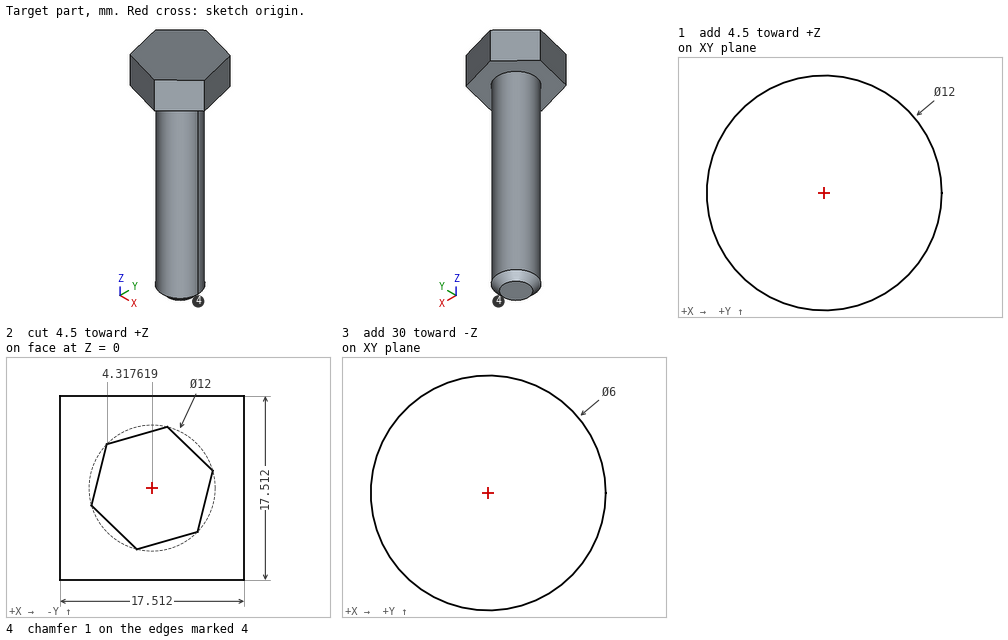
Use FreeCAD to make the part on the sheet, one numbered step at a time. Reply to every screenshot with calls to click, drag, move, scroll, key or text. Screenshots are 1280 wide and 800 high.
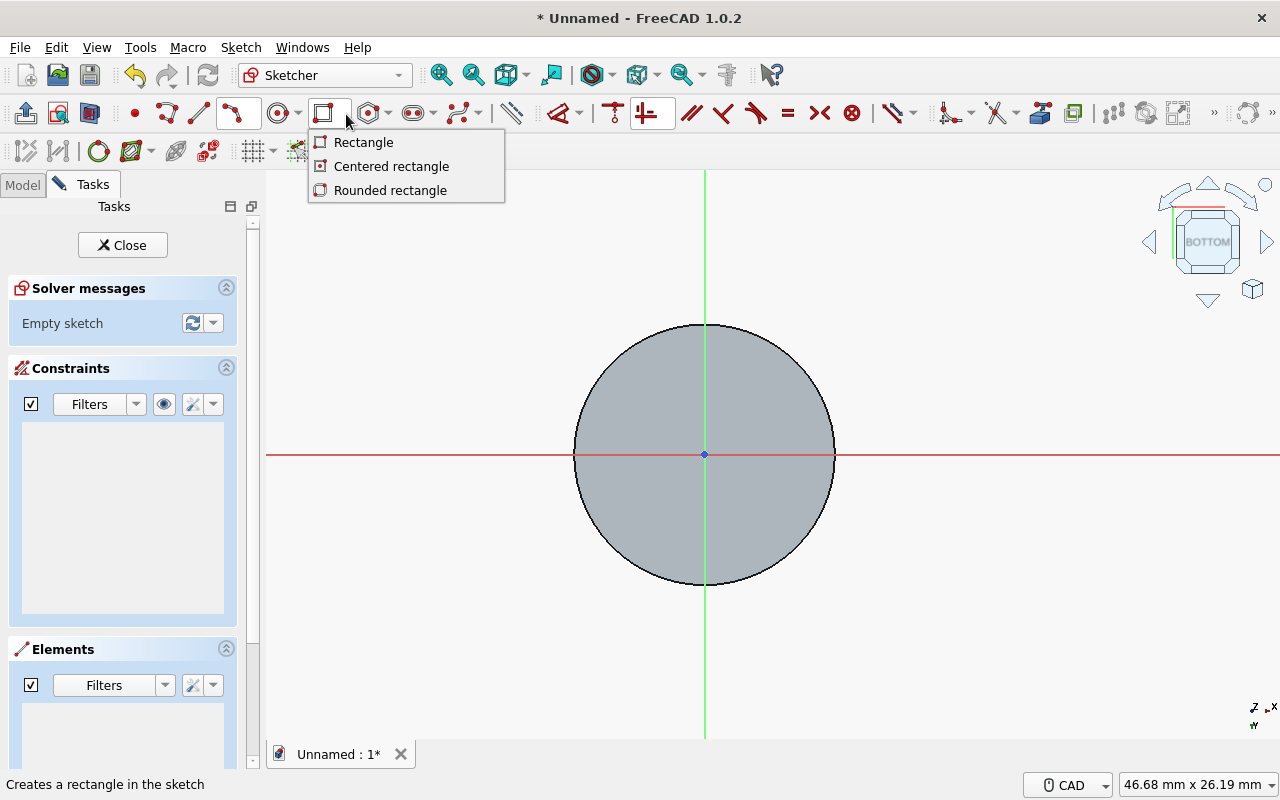
click(406, 166)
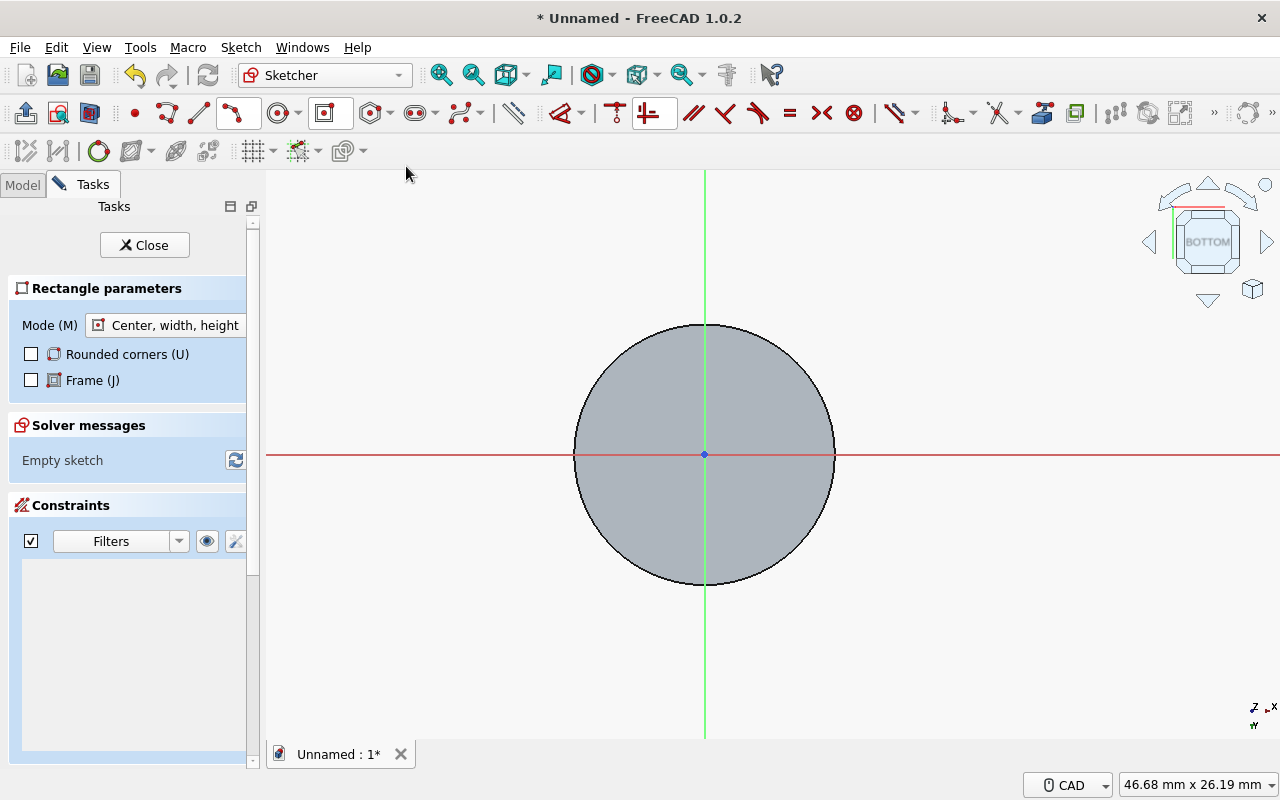
click(705, 455)
click(895, 265)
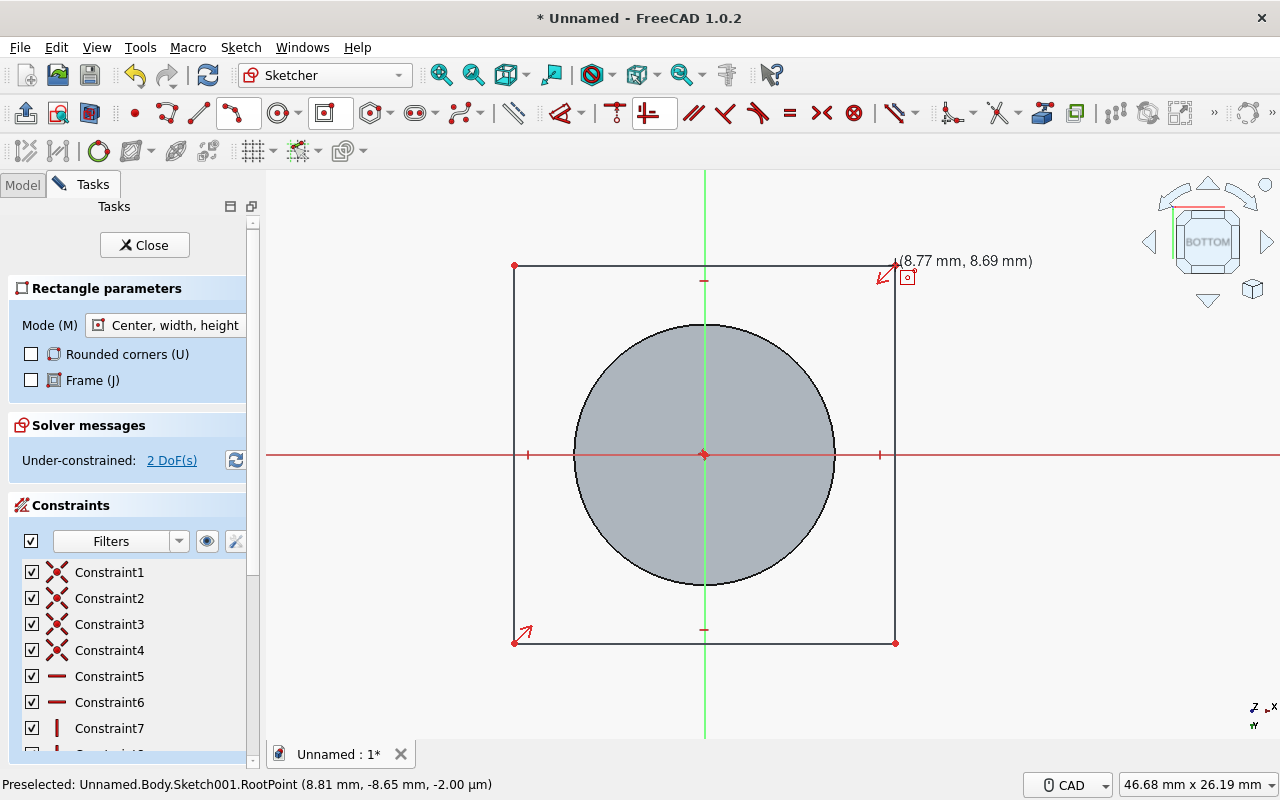
click(370, 114)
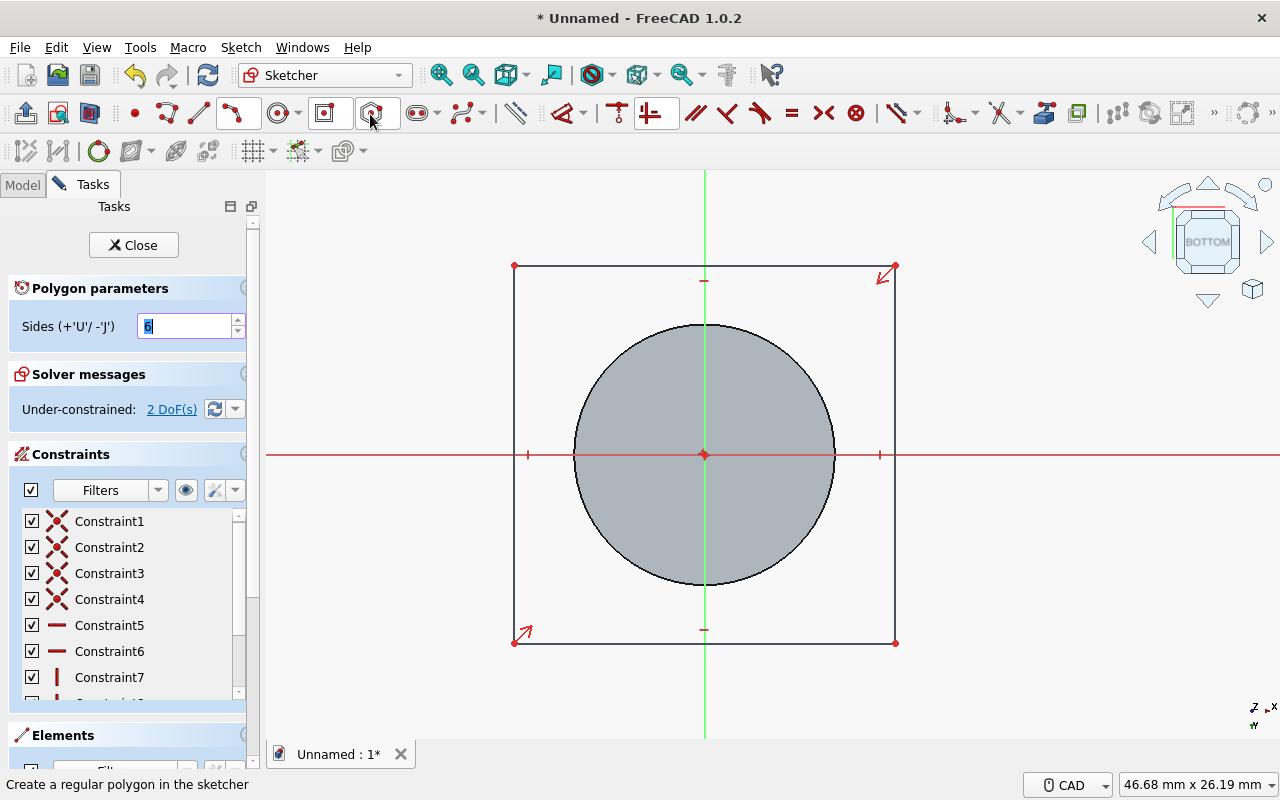
click(705, 455)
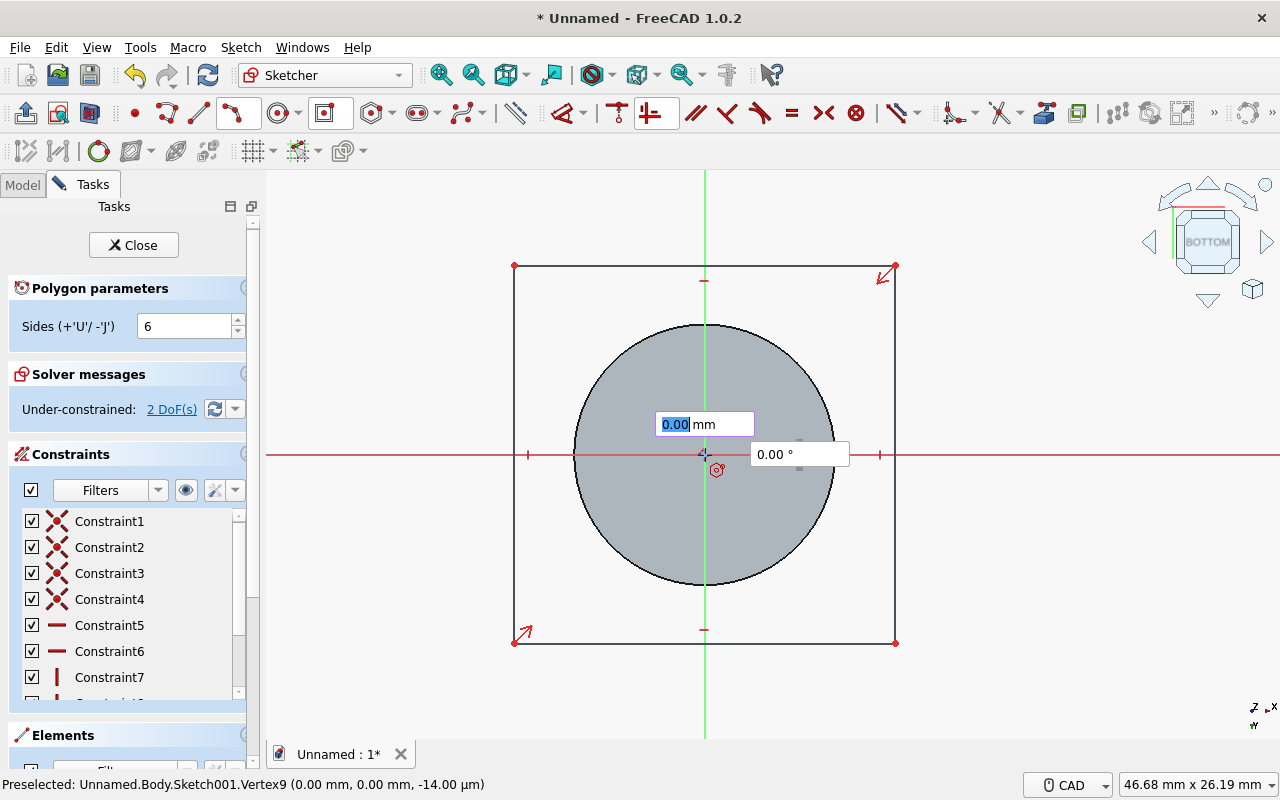
click(611, 364)
right_click(611, 364)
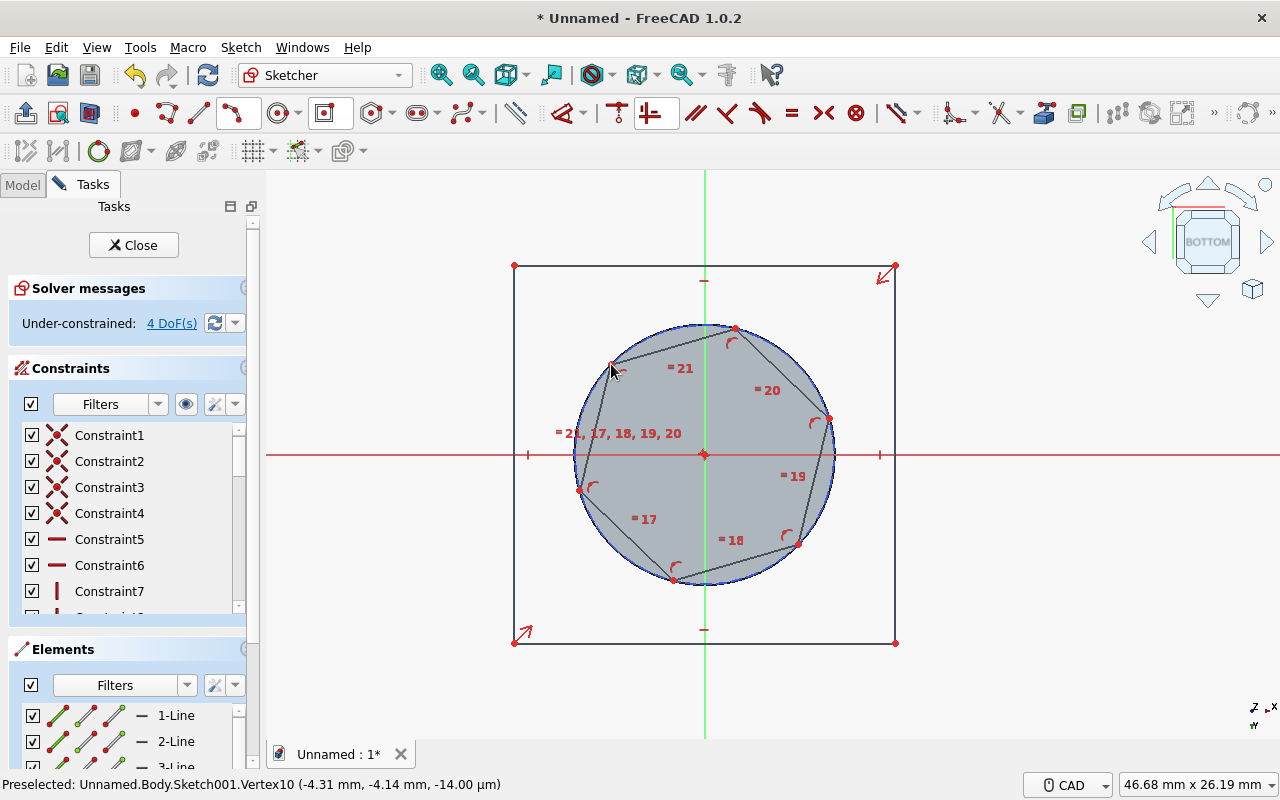
click(796, 363)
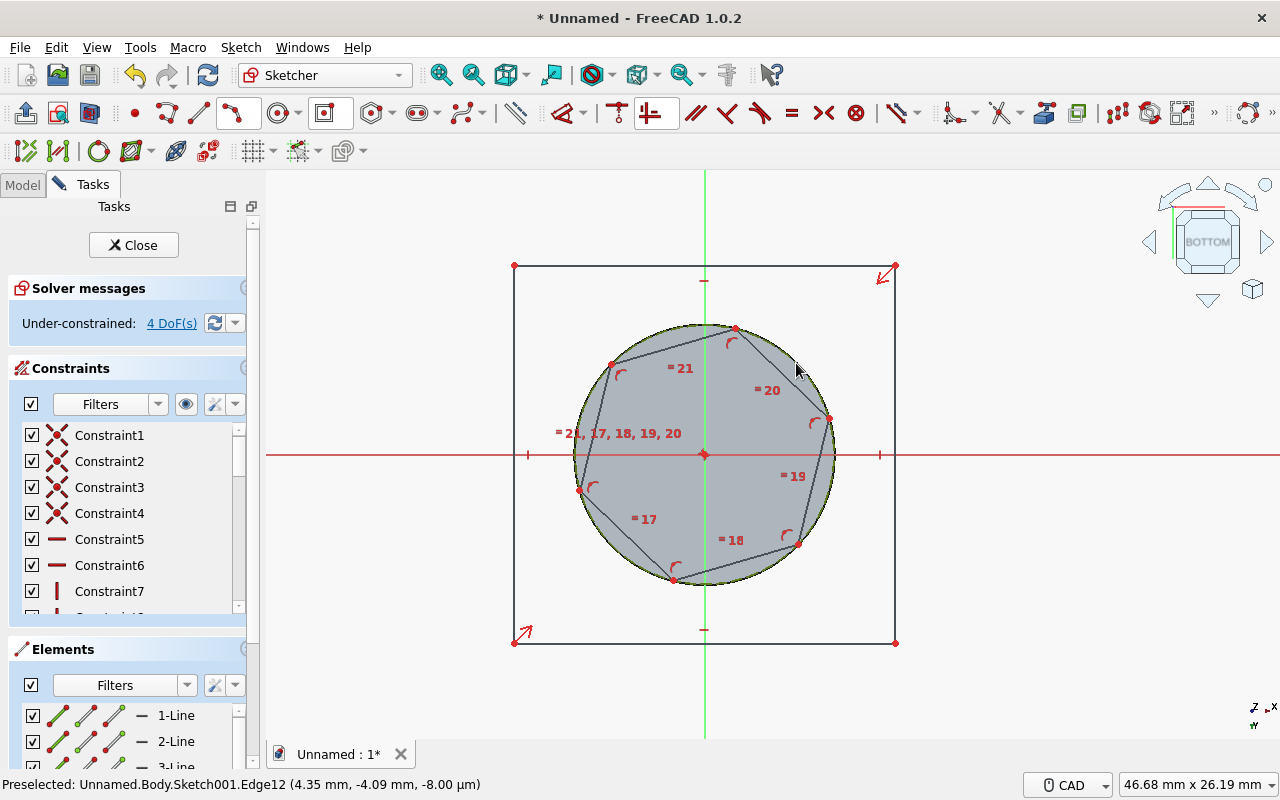
key(k)
key(o)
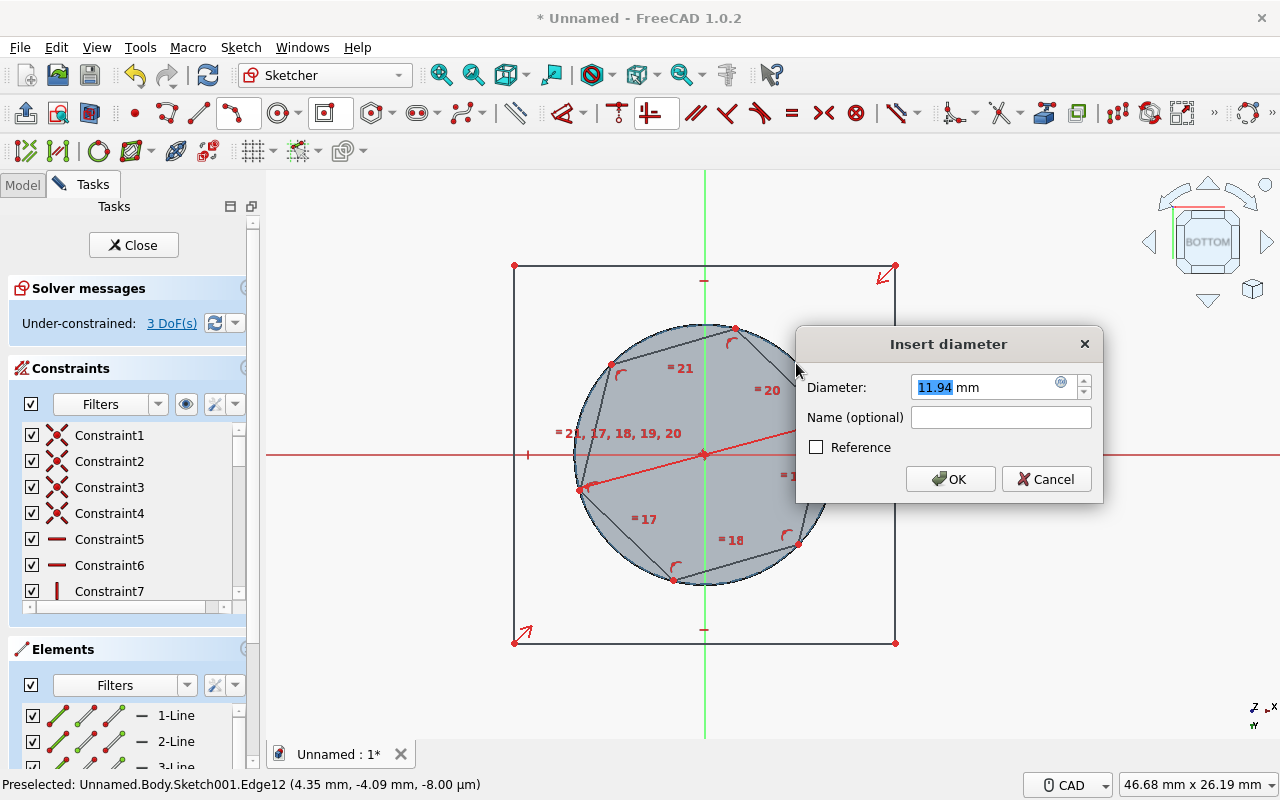
text(12)
key(Return)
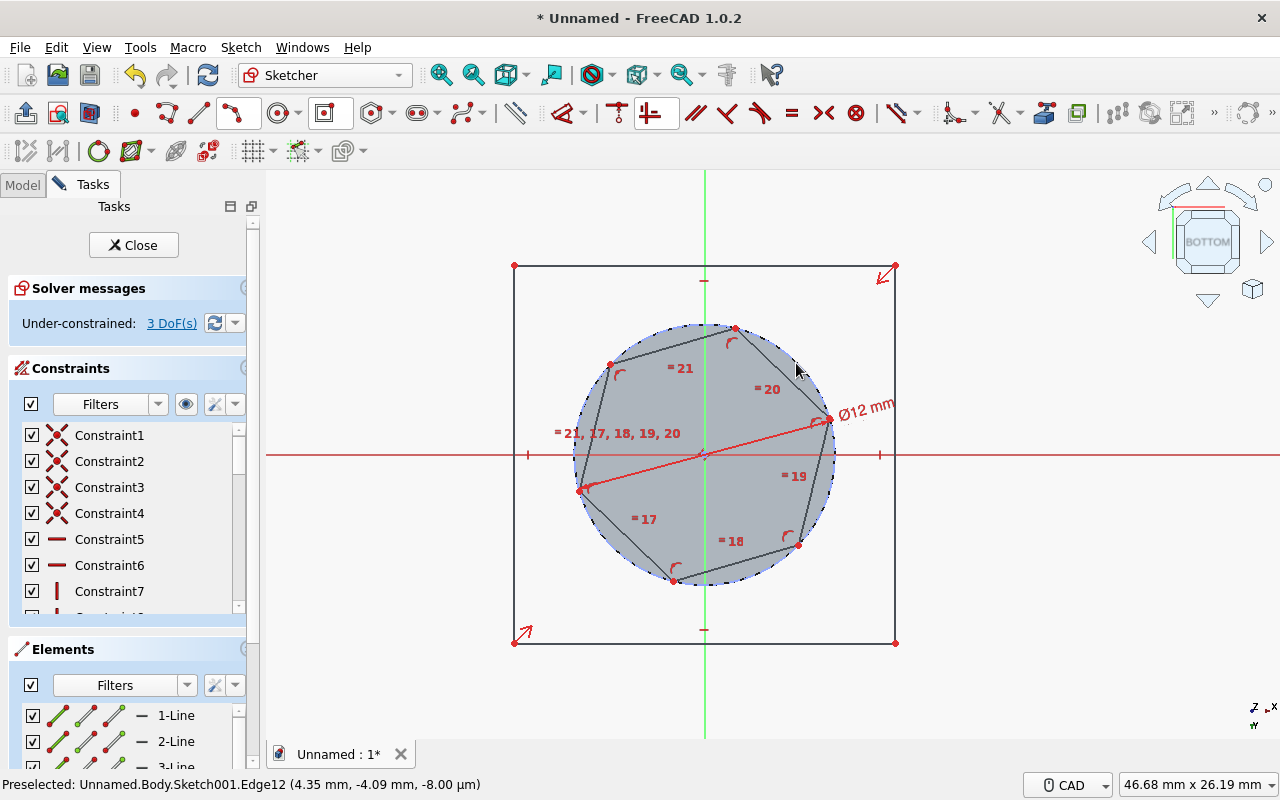
click(628, 644)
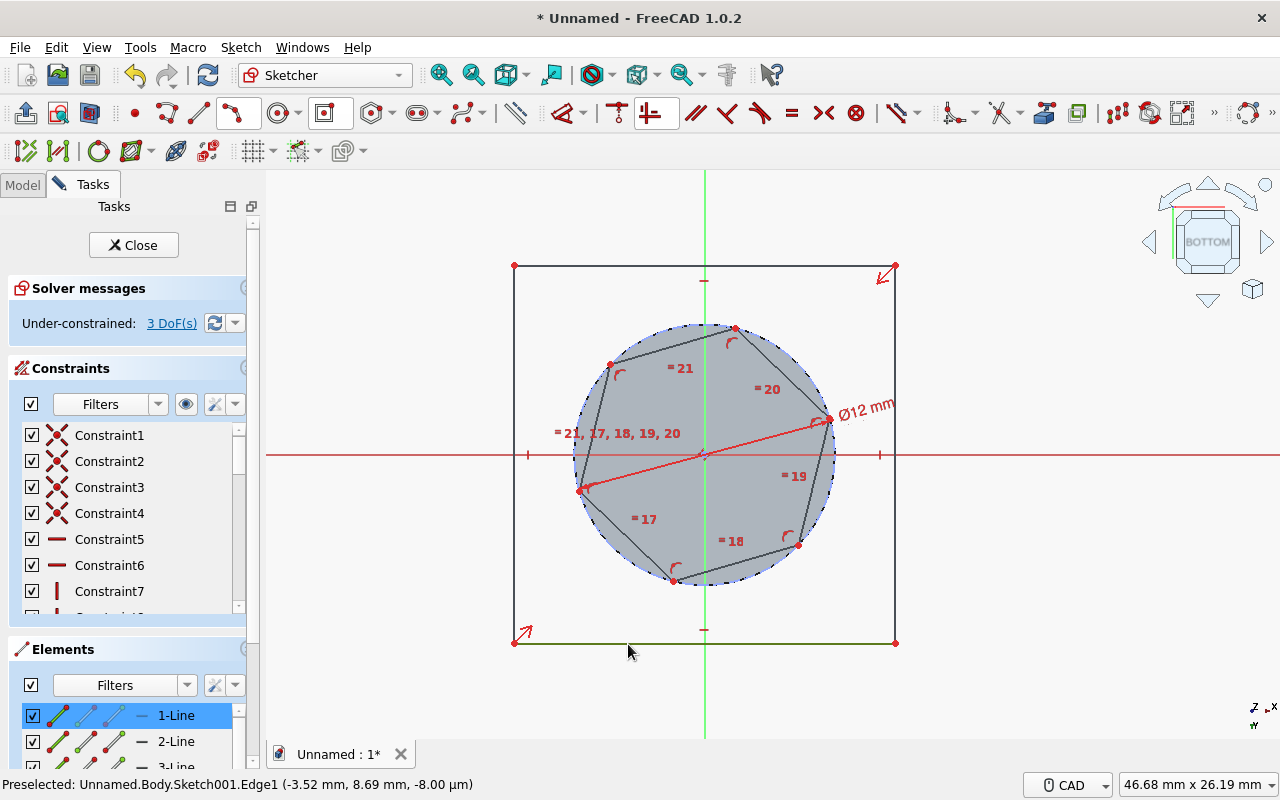
key(l)